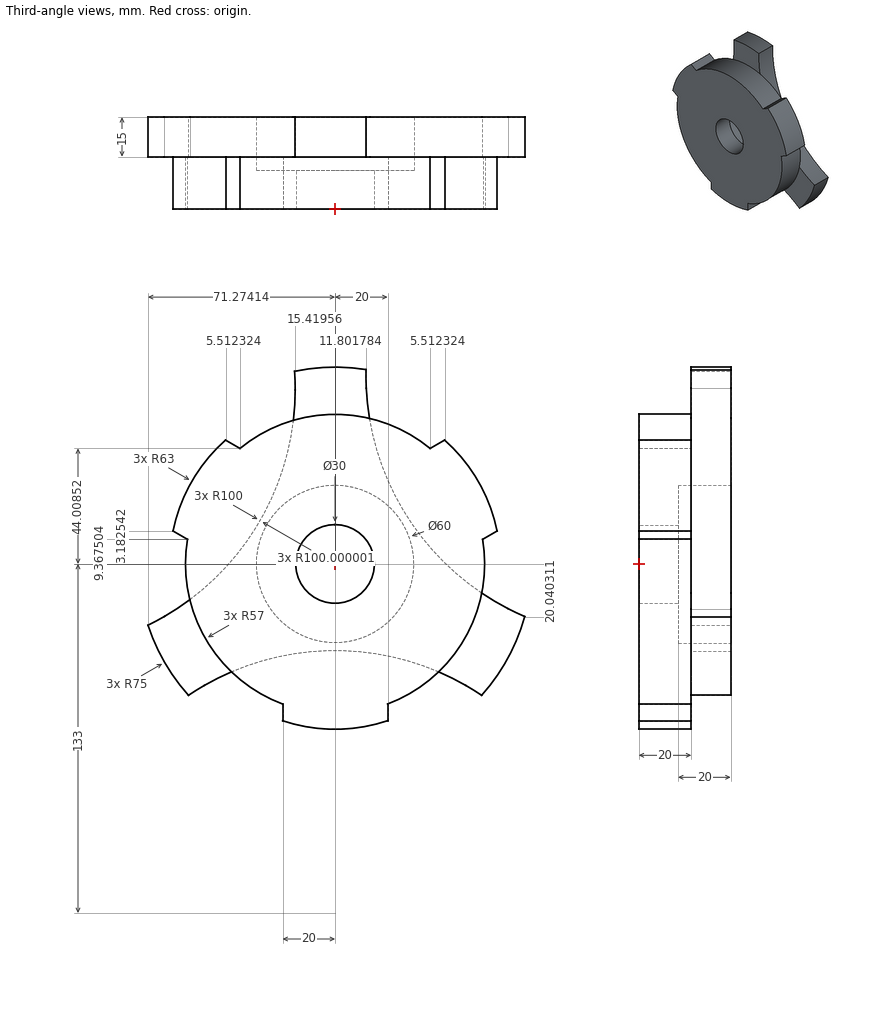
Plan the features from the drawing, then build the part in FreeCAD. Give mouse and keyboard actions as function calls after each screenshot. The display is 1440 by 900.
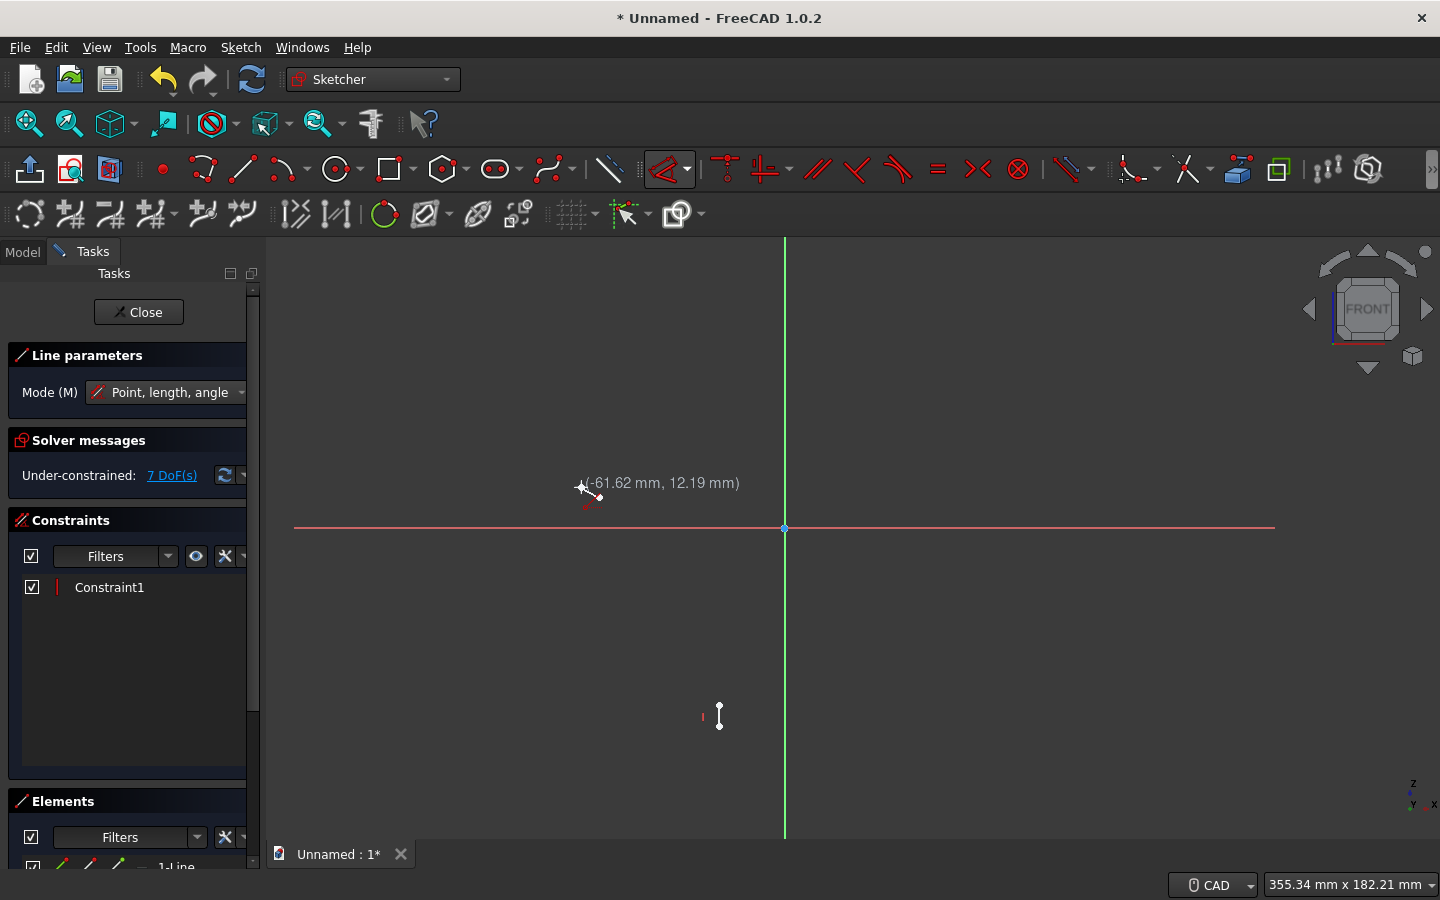
click(647, 372)
click(665, 383)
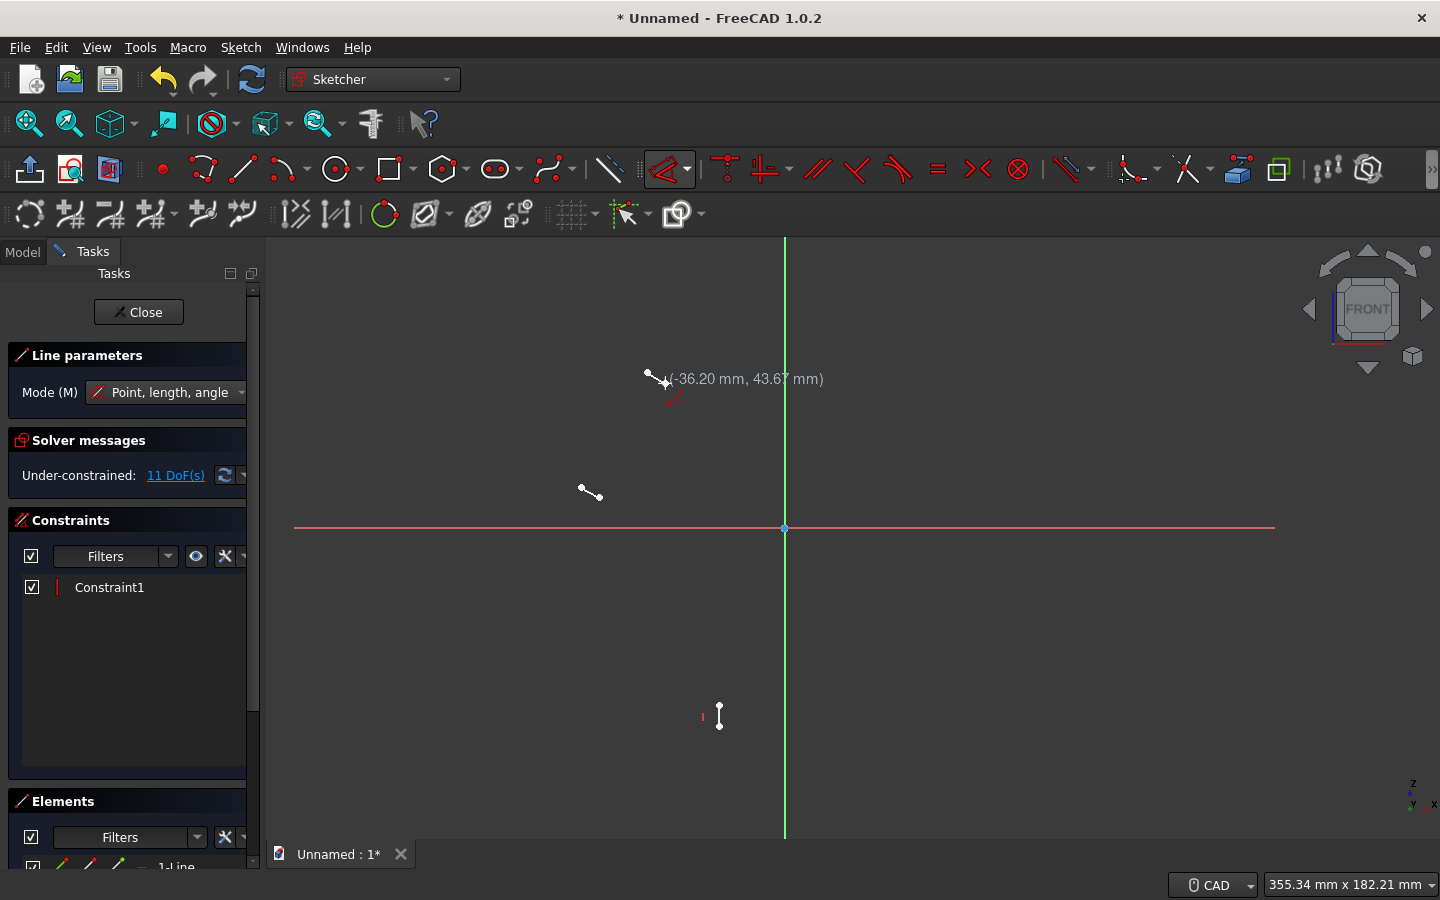
click(904, 383)
click(922, 372)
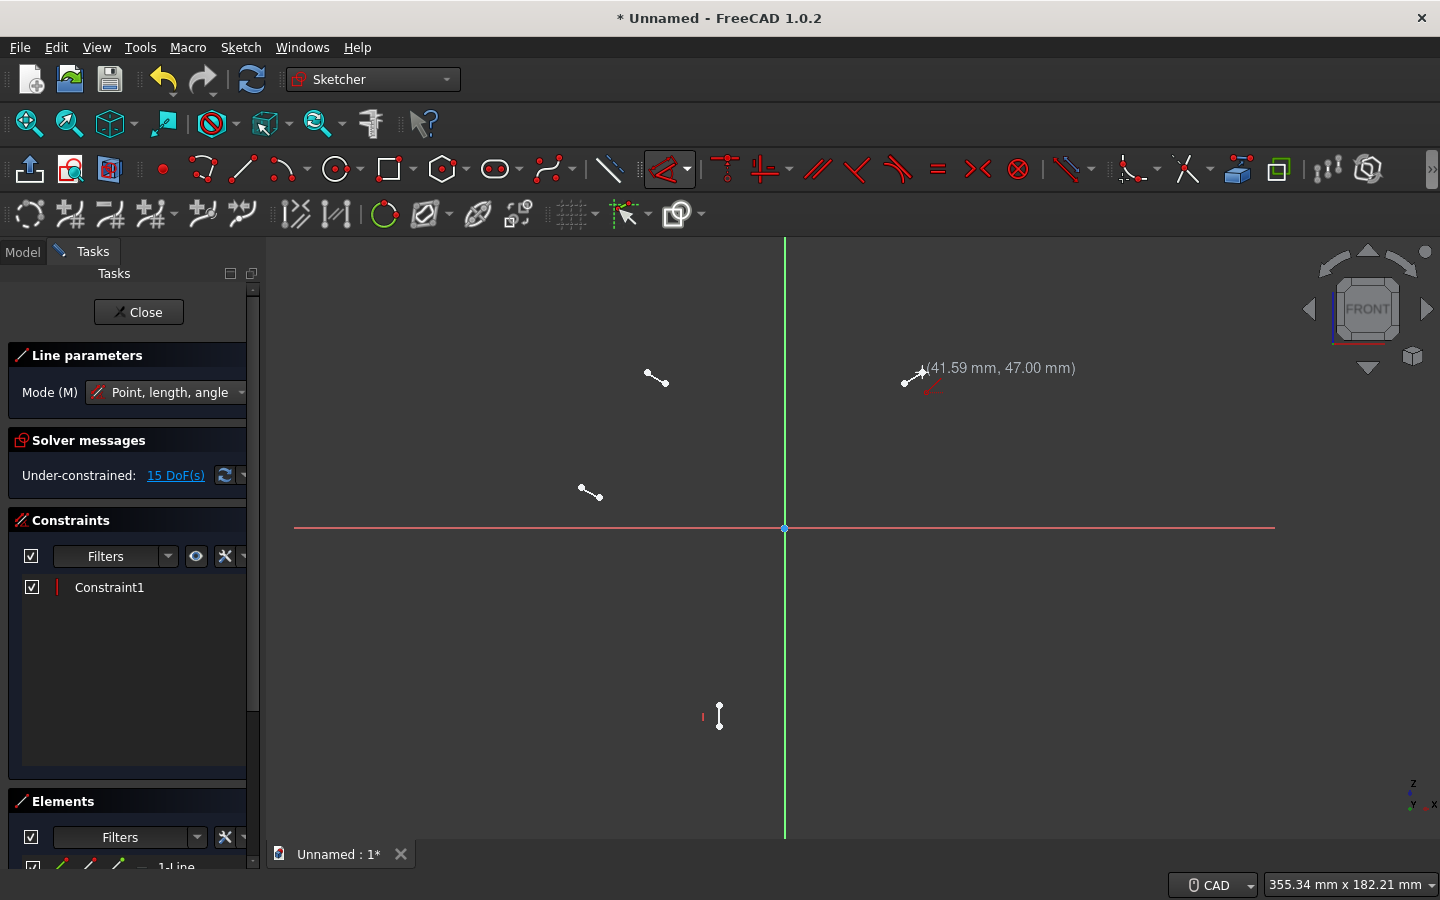
click(989, 487)
click(970, 497)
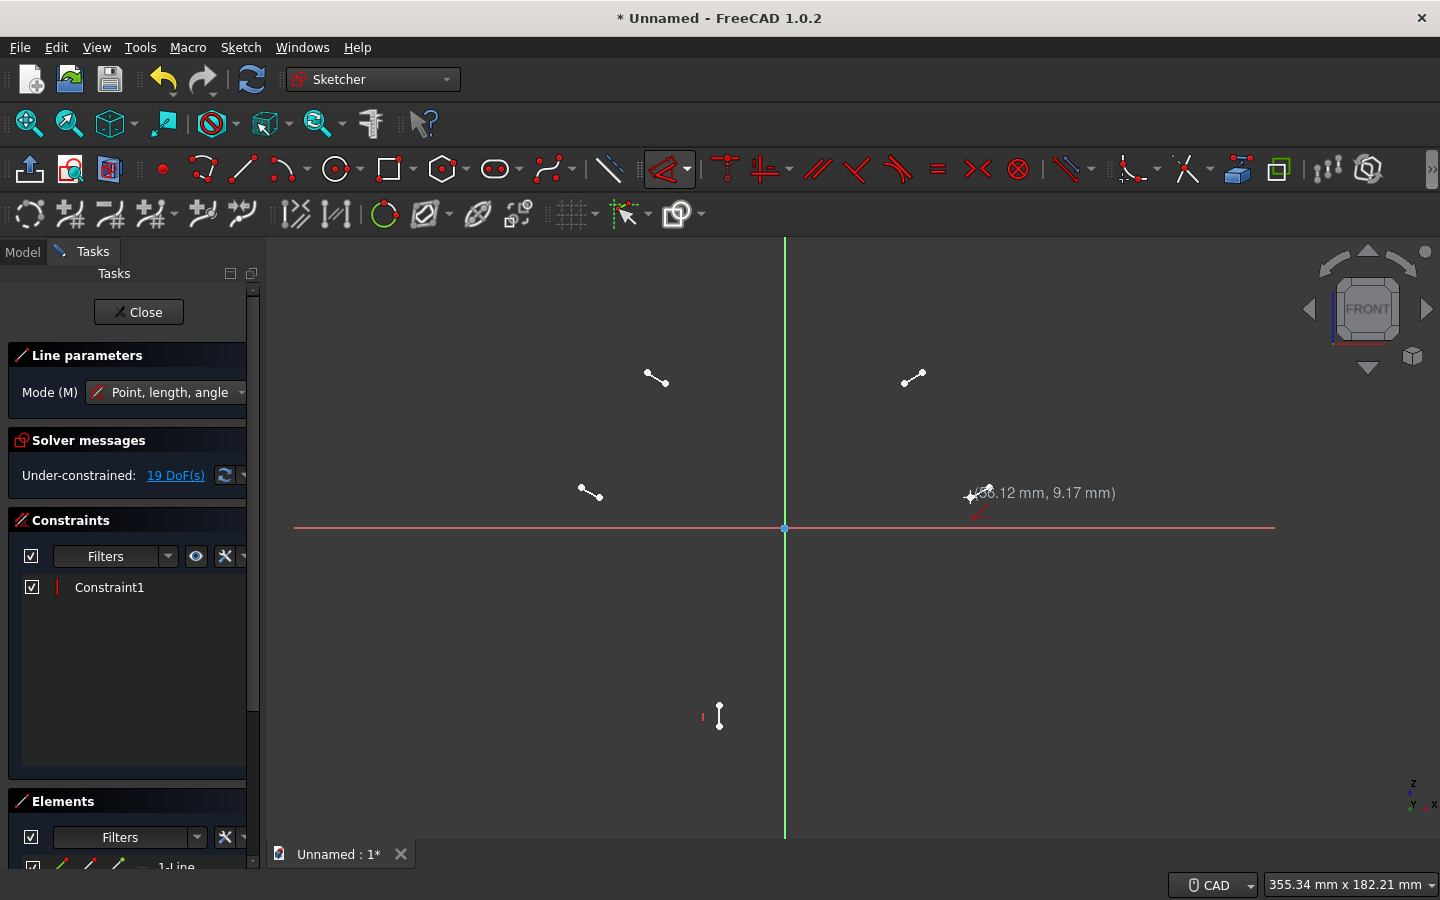
click(851, 705)
click(851, 726)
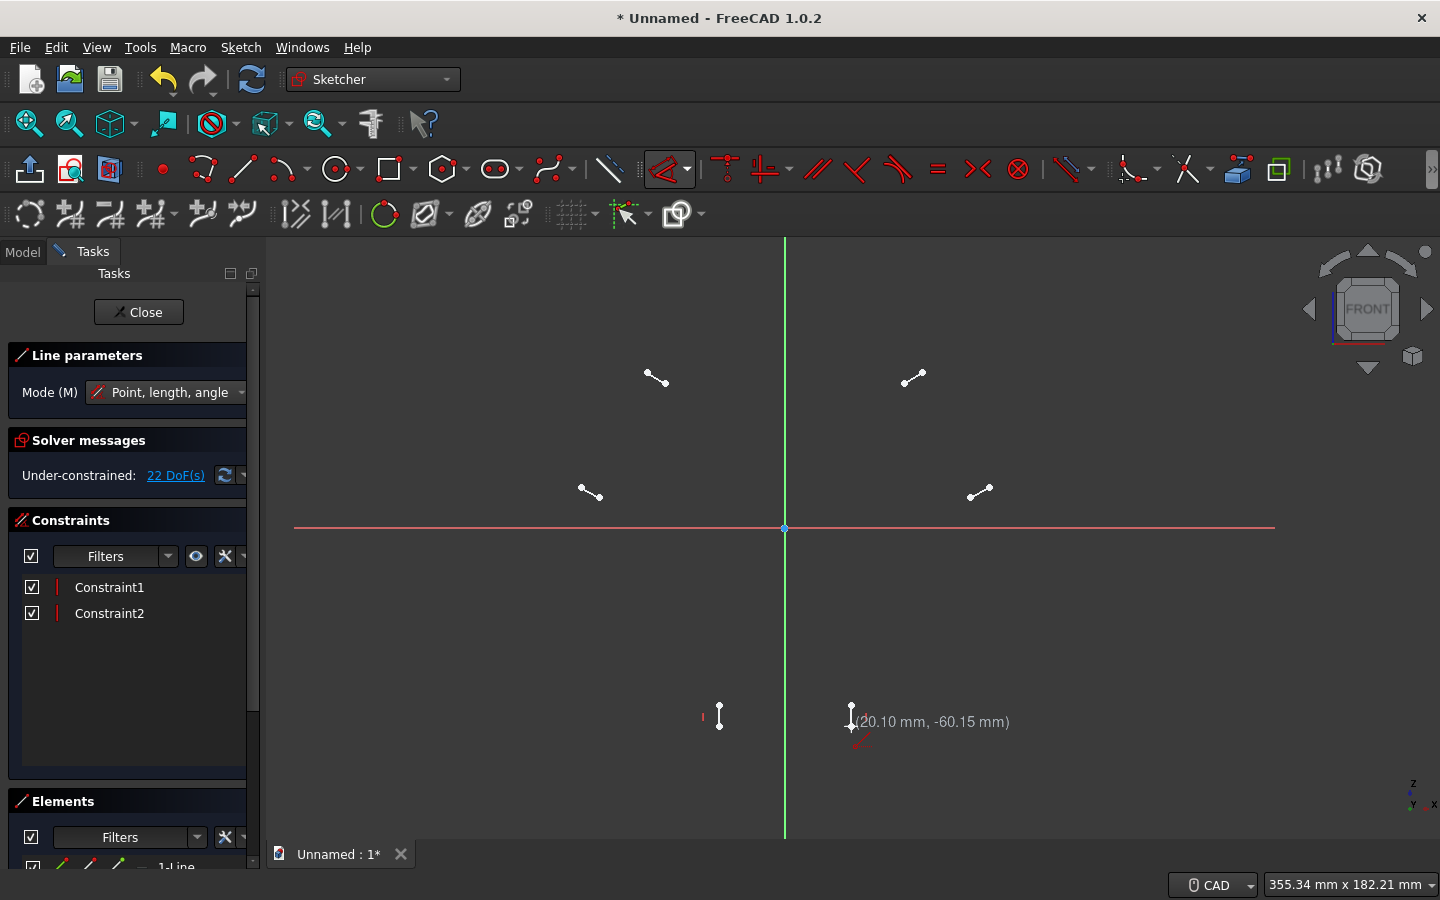
key(g)
key(3)
key(a)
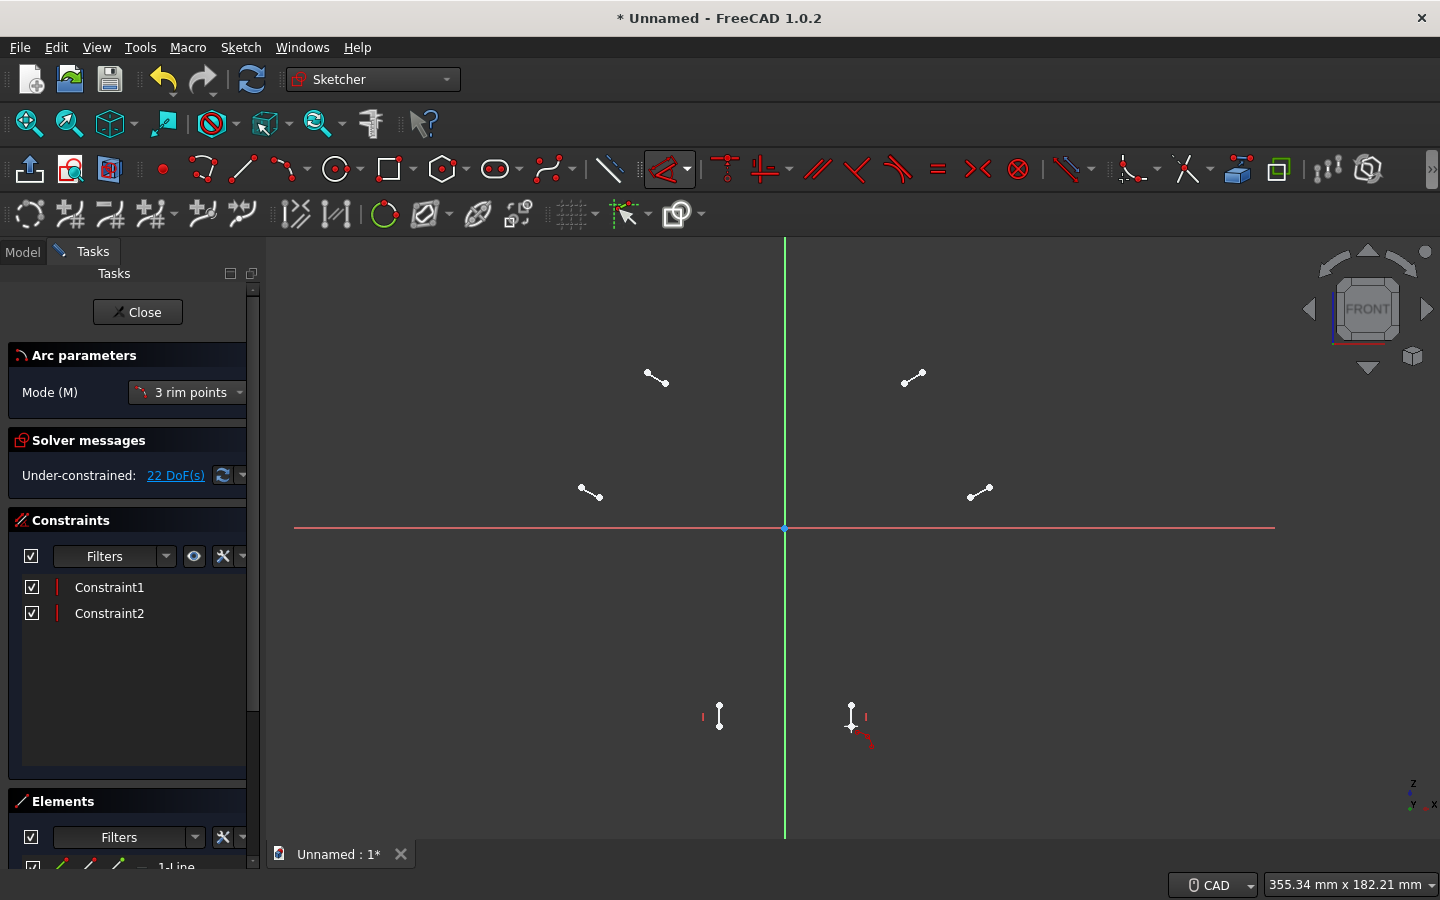
scroll(719, 705, up, 3)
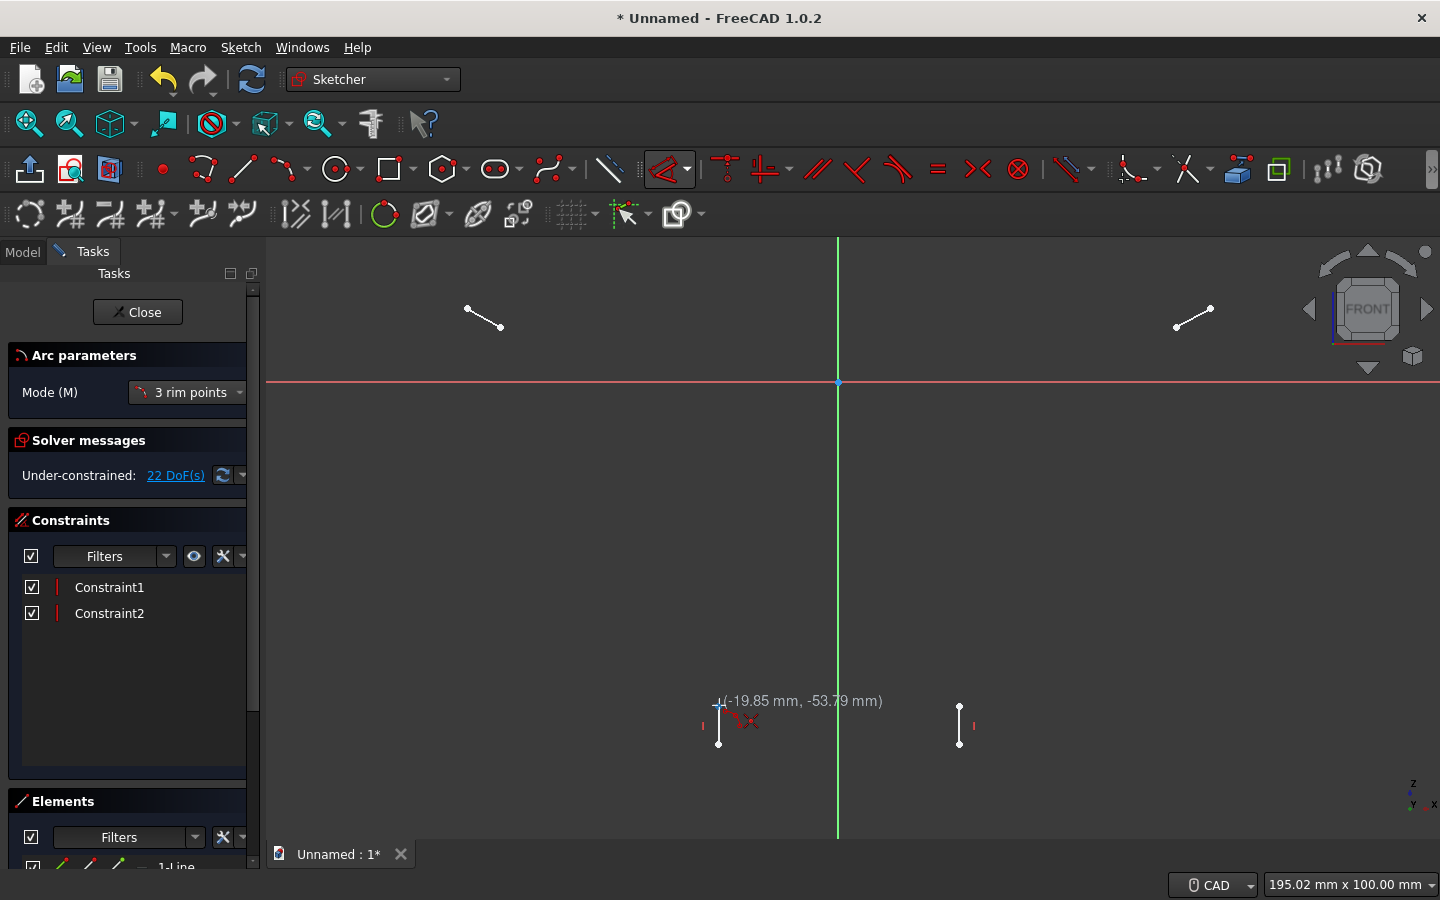
click(719, 706)
click(500, 327)
click(541, 554)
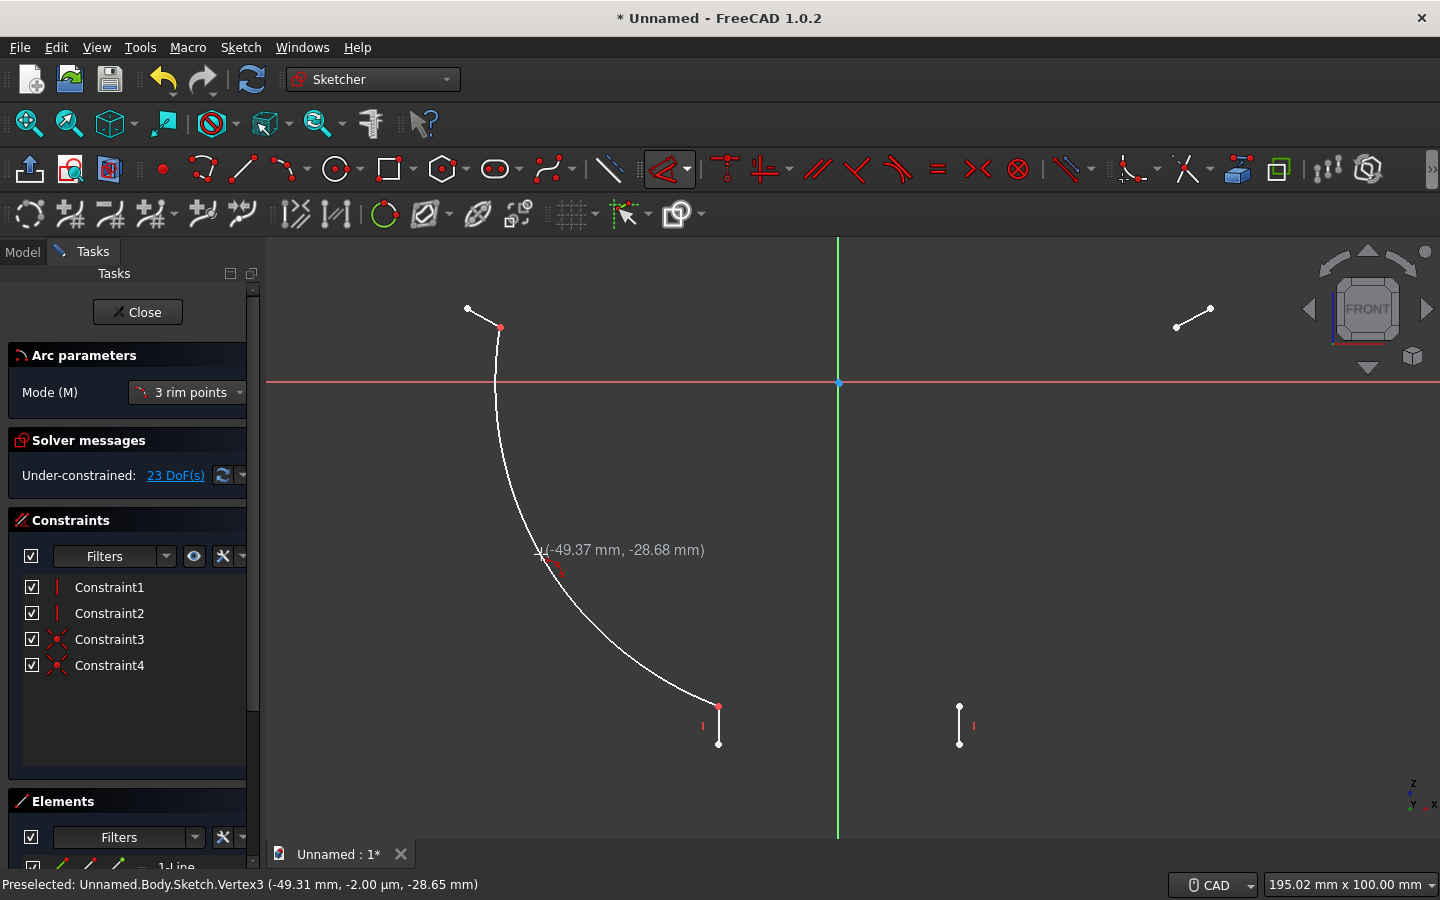
click(467, 309)